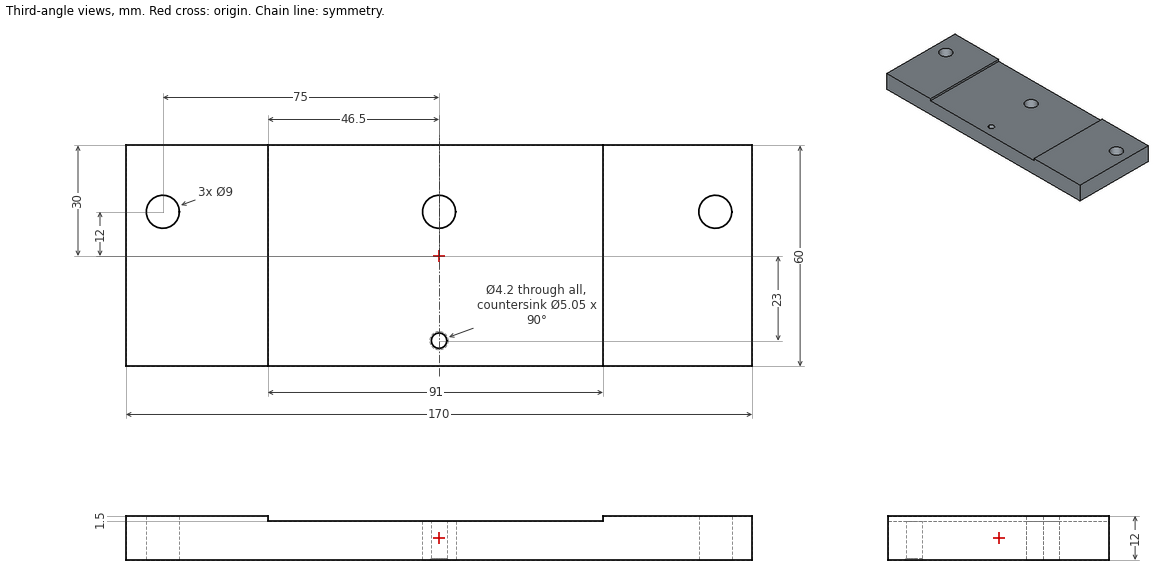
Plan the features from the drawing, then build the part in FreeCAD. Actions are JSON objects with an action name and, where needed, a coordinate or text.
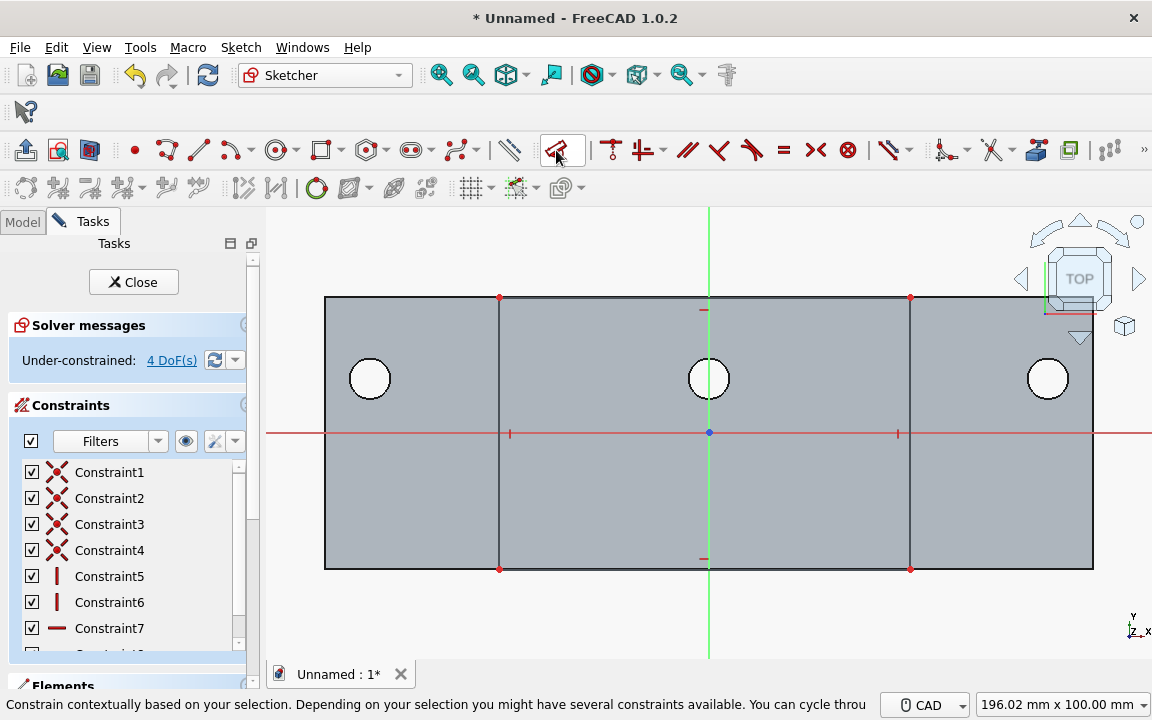
{"action": "left_click", "coordinate": [499, 380]}
{"action": "left_click", "coordinate": [465, 371]}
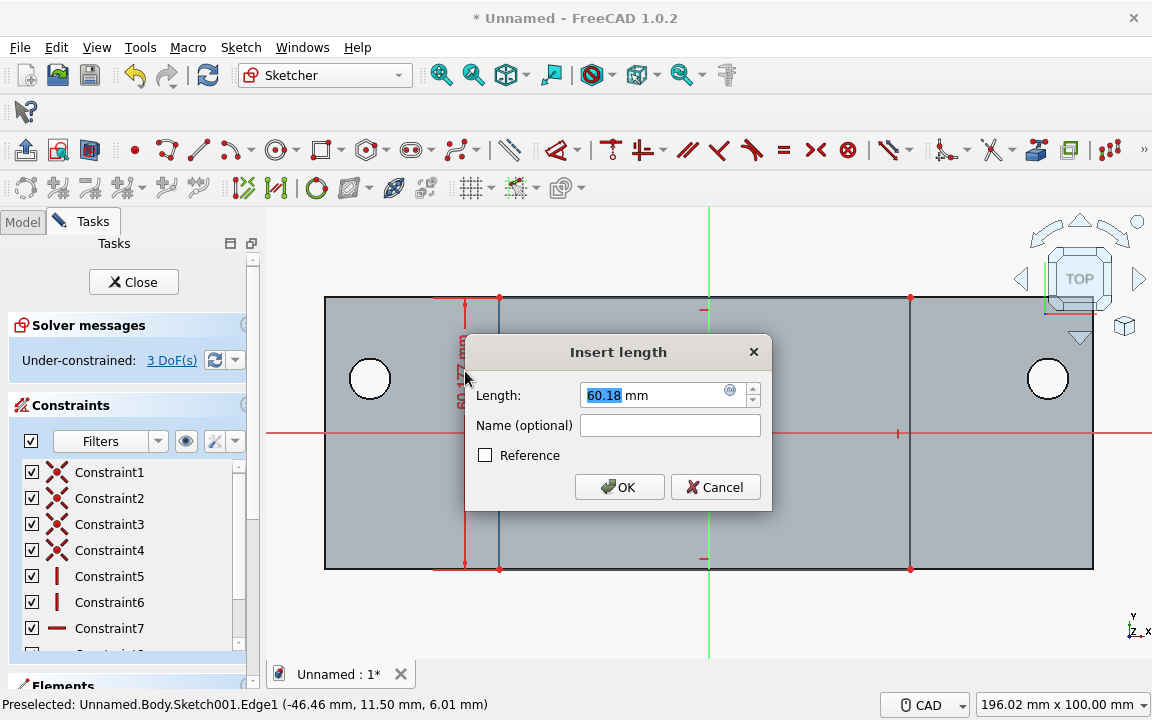
{"action": "type", "text": "60"}
{"action": "key", "text": "Return"}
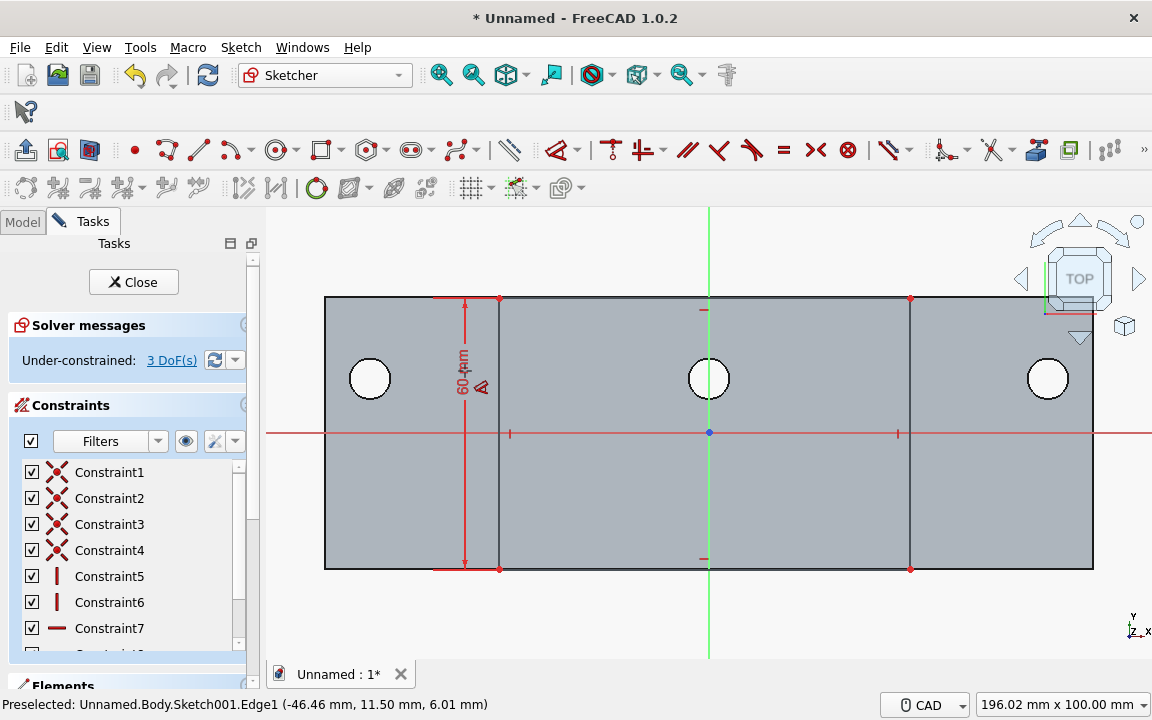
{"action": "left_click", "coordinate": [622, 570]}
{"action": "left_click", "coordinate": [610, 604]}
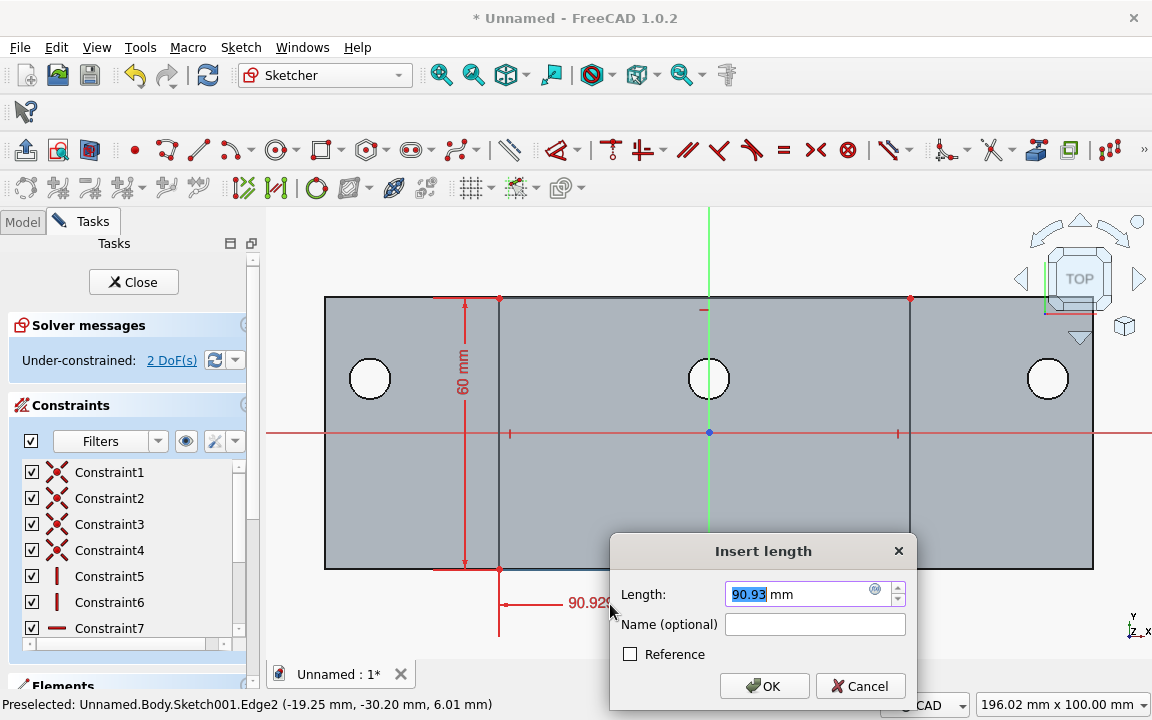
{"action": "type", "text": "91"}
{"action": "key", "text": "Return"}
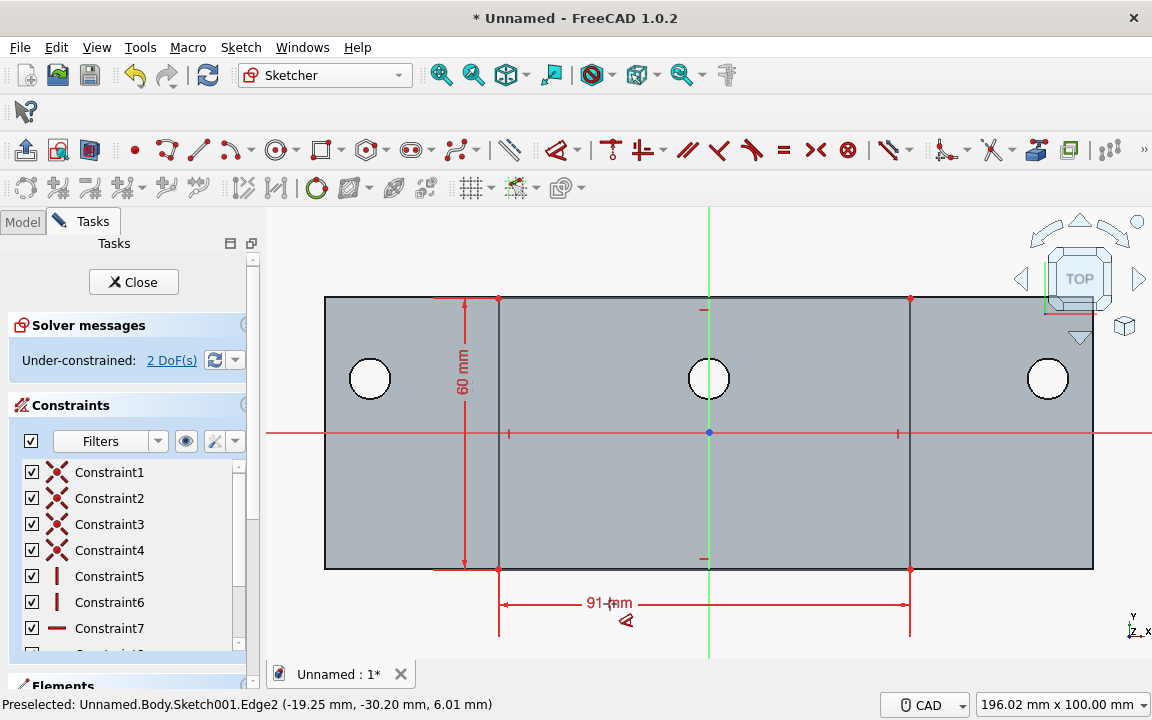
{"action": "left_click", "coordinate": [499, 298]}
{"action": "left_click", "coordinate": [465, 335]}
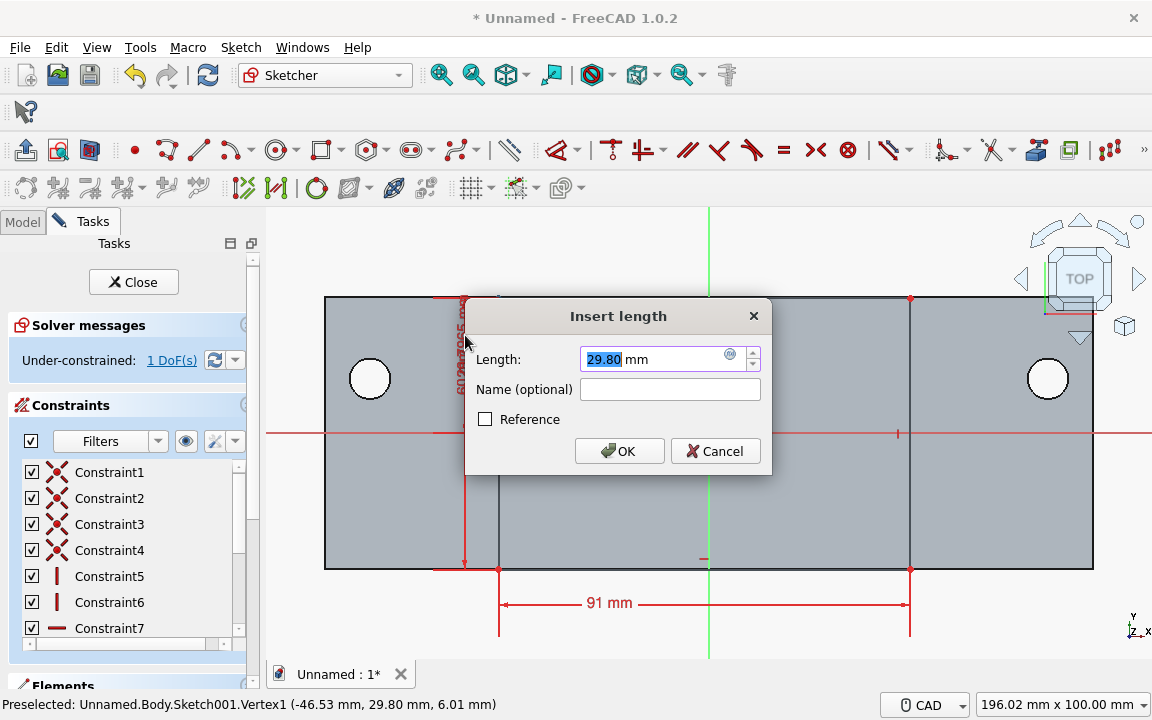
{"action": "type", "text": "30"}
{"action": "key", "text": "Return"}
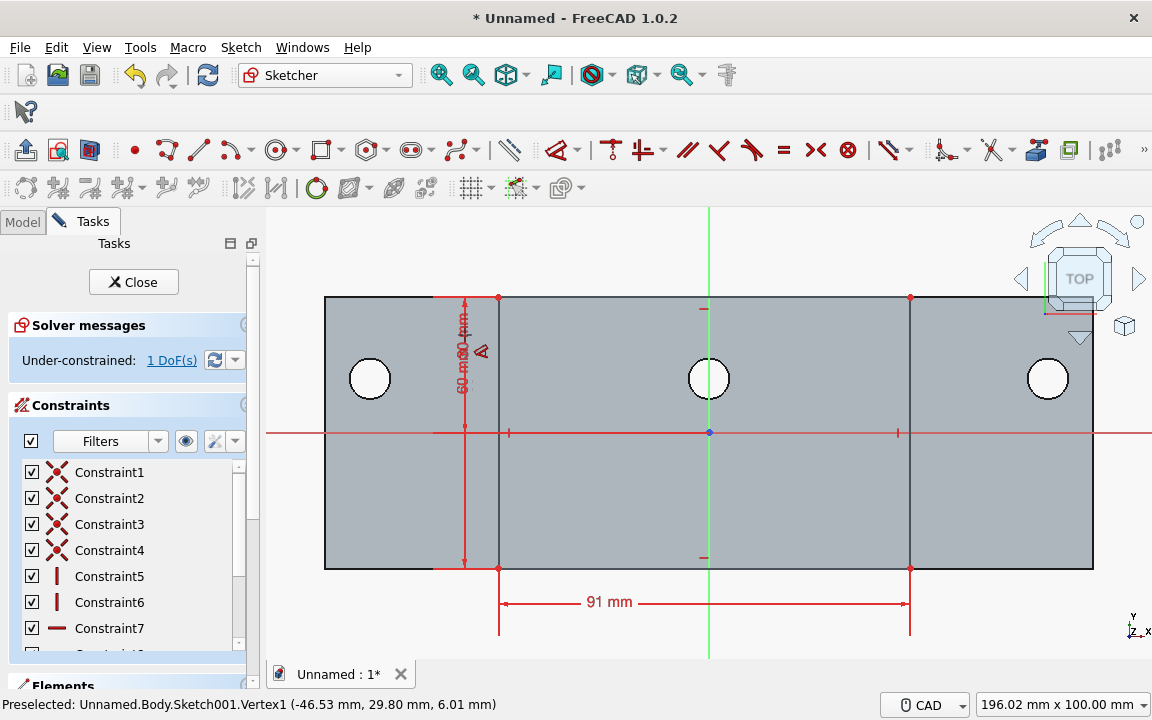
{"action": "left_click", "coordinate": [499, 297]}
{"action": "left_click", "coordinate": [604, 263]}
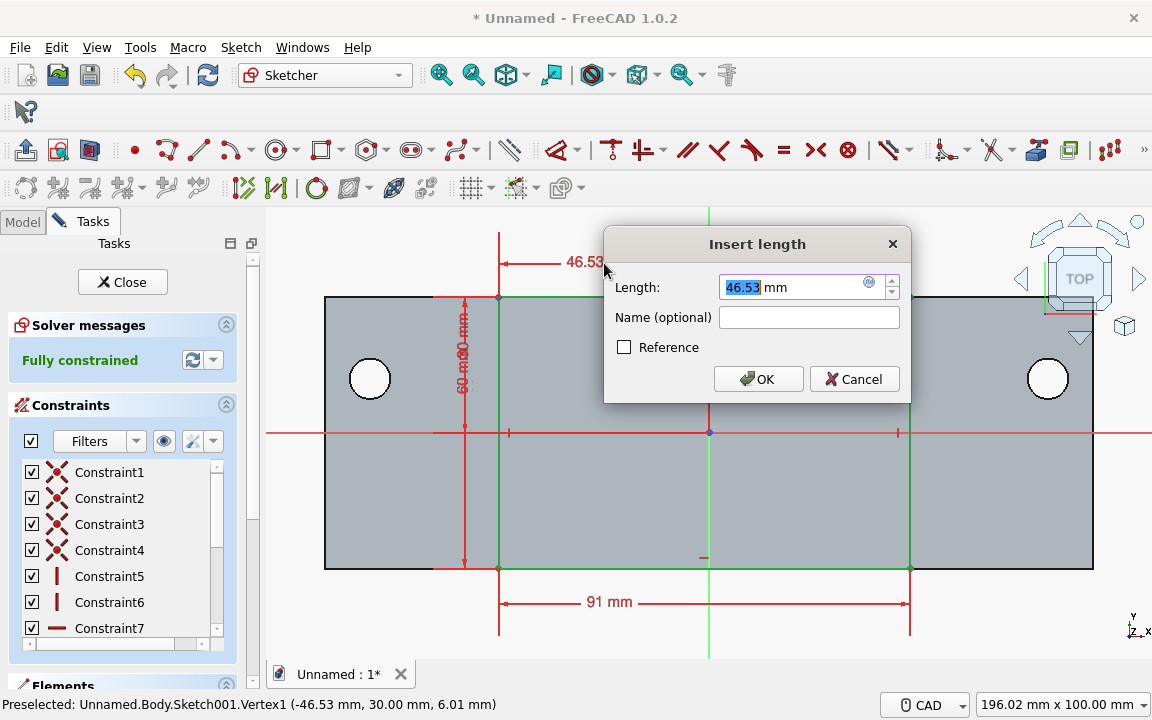
{"action": "type", "text": "46.5"}
{"action": "key", "text": "Return"}
{"action": "key", "text": "Escape"}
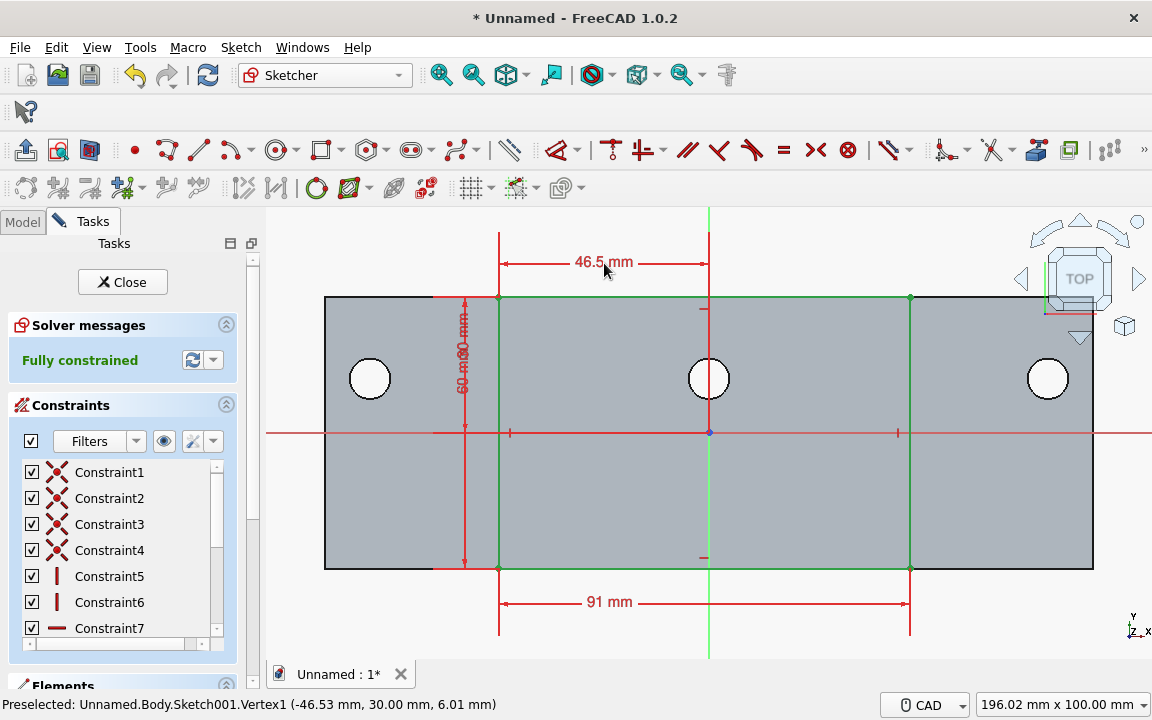
{"action": "left_click", "coordinate": [123, 282]}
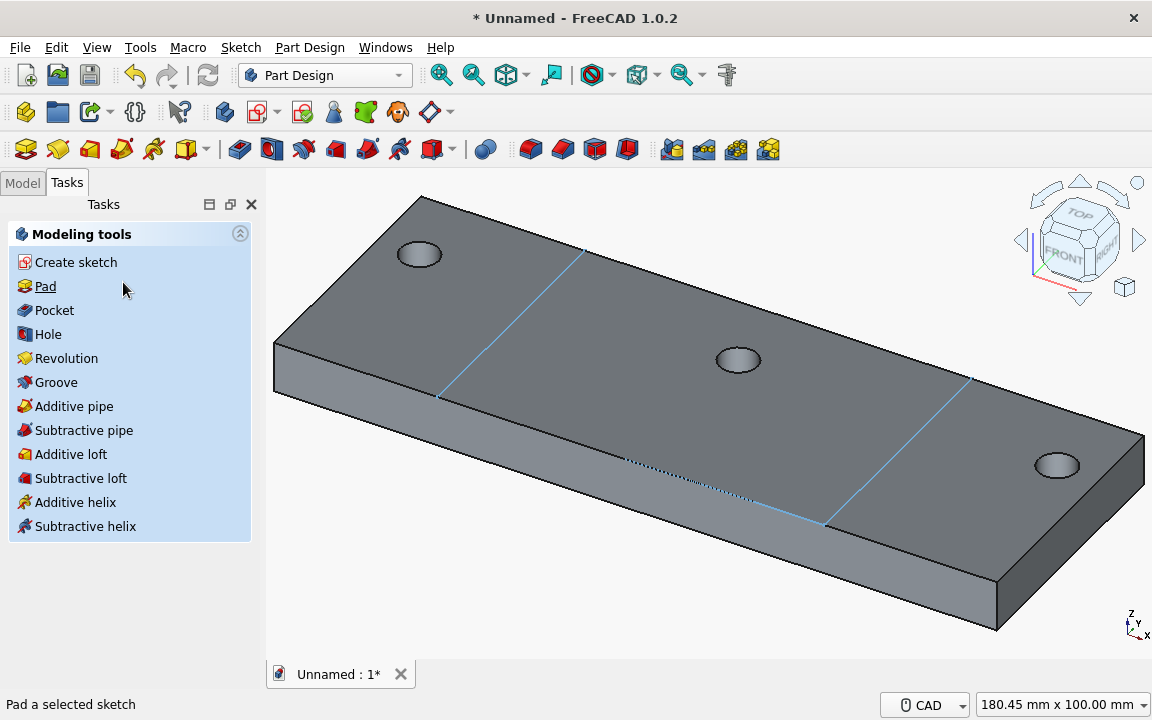
{"action": "left_click", "coordinate": [240, 150]}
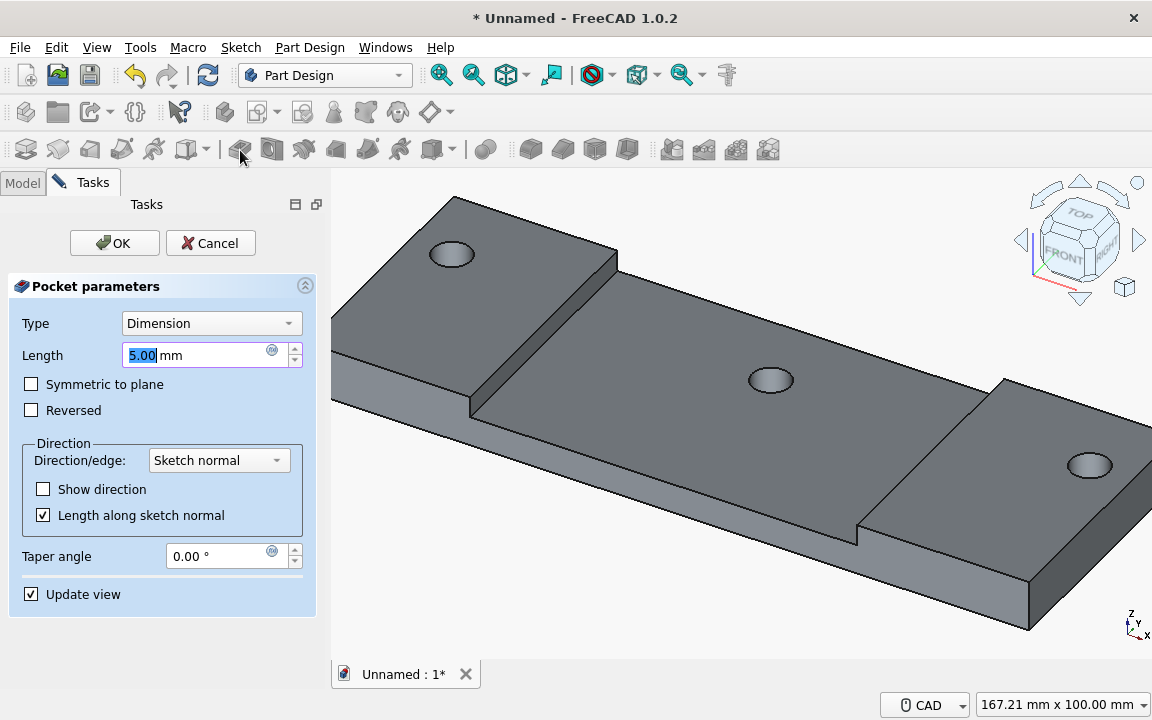
{"action": "type", "text": "1.5"}
{"action": "key", "text": "Tab"}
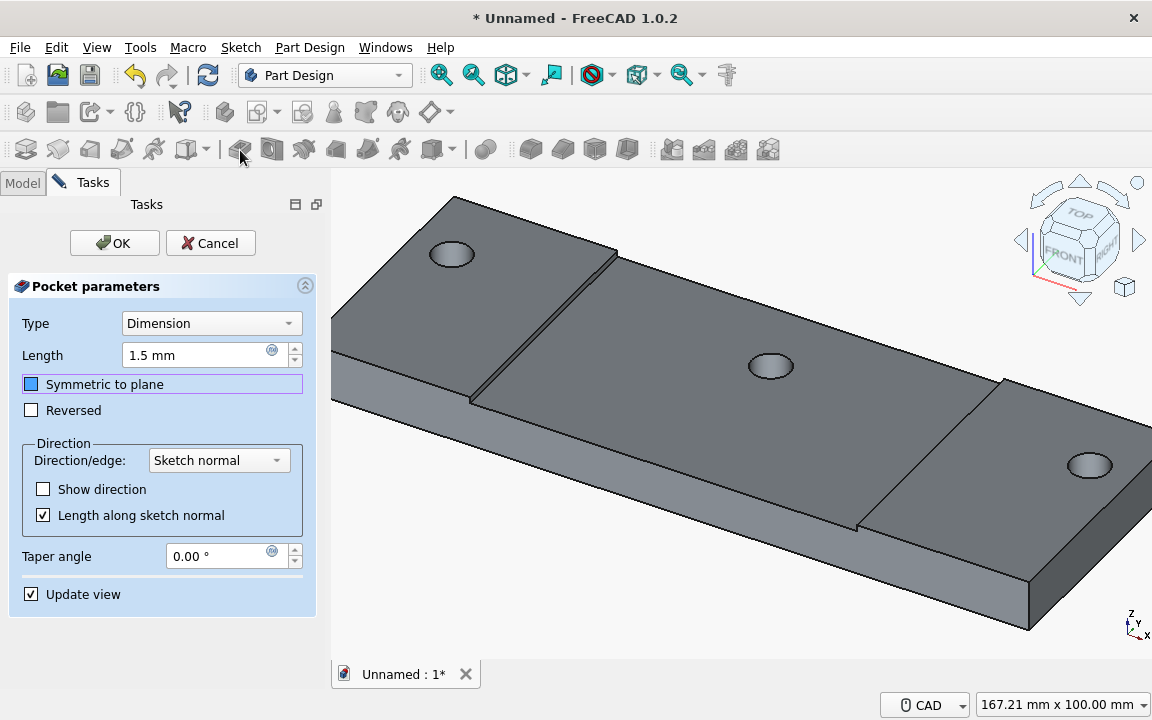
{"action": "left_click", "coordinate": [115, 243]}